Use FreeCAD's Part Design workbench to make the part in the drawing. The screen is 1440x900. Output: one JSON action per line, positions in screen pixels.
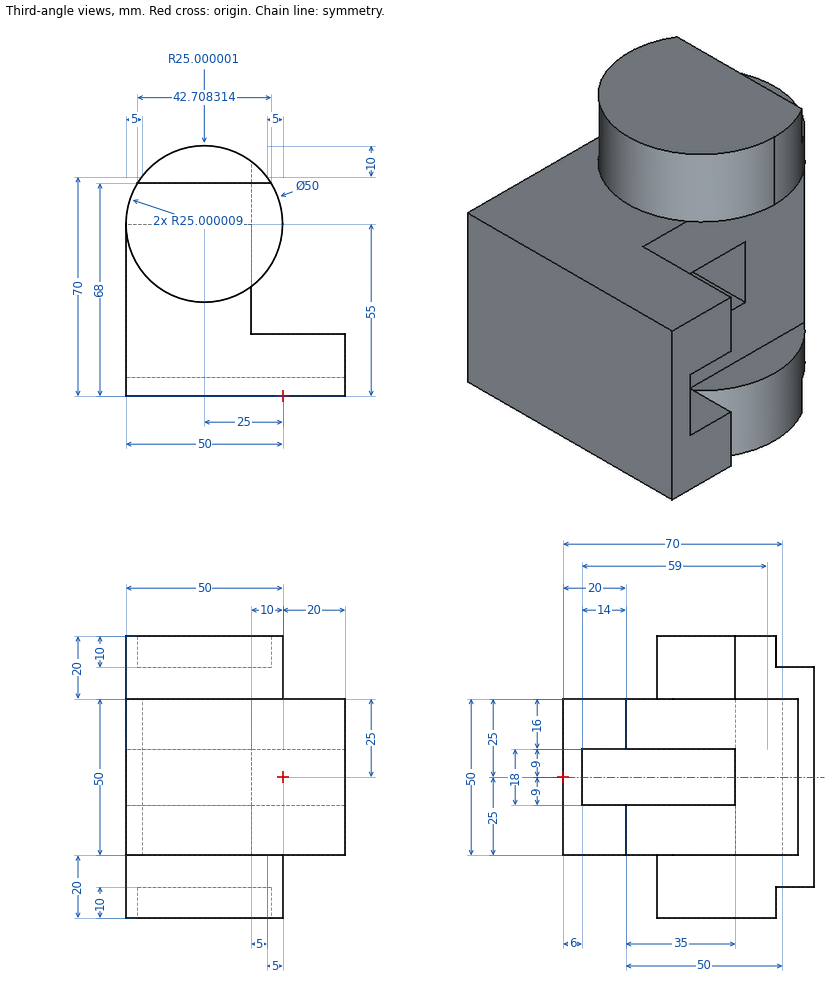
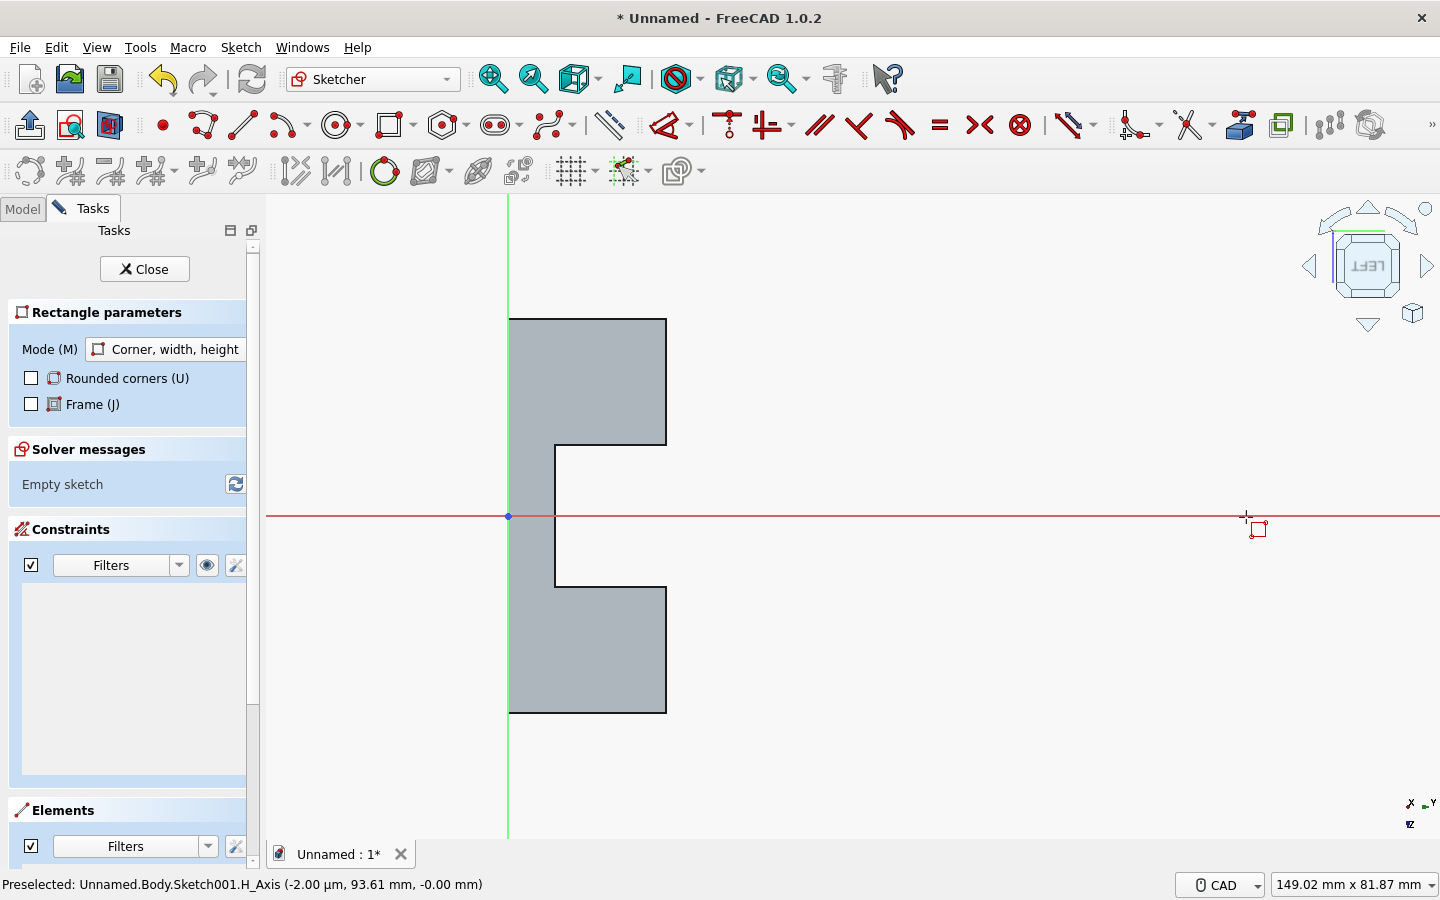
{"action": "left_click", "coordinate": [508, 319]}
{"action": "mouse_move", "coordinate": [1060, 713]}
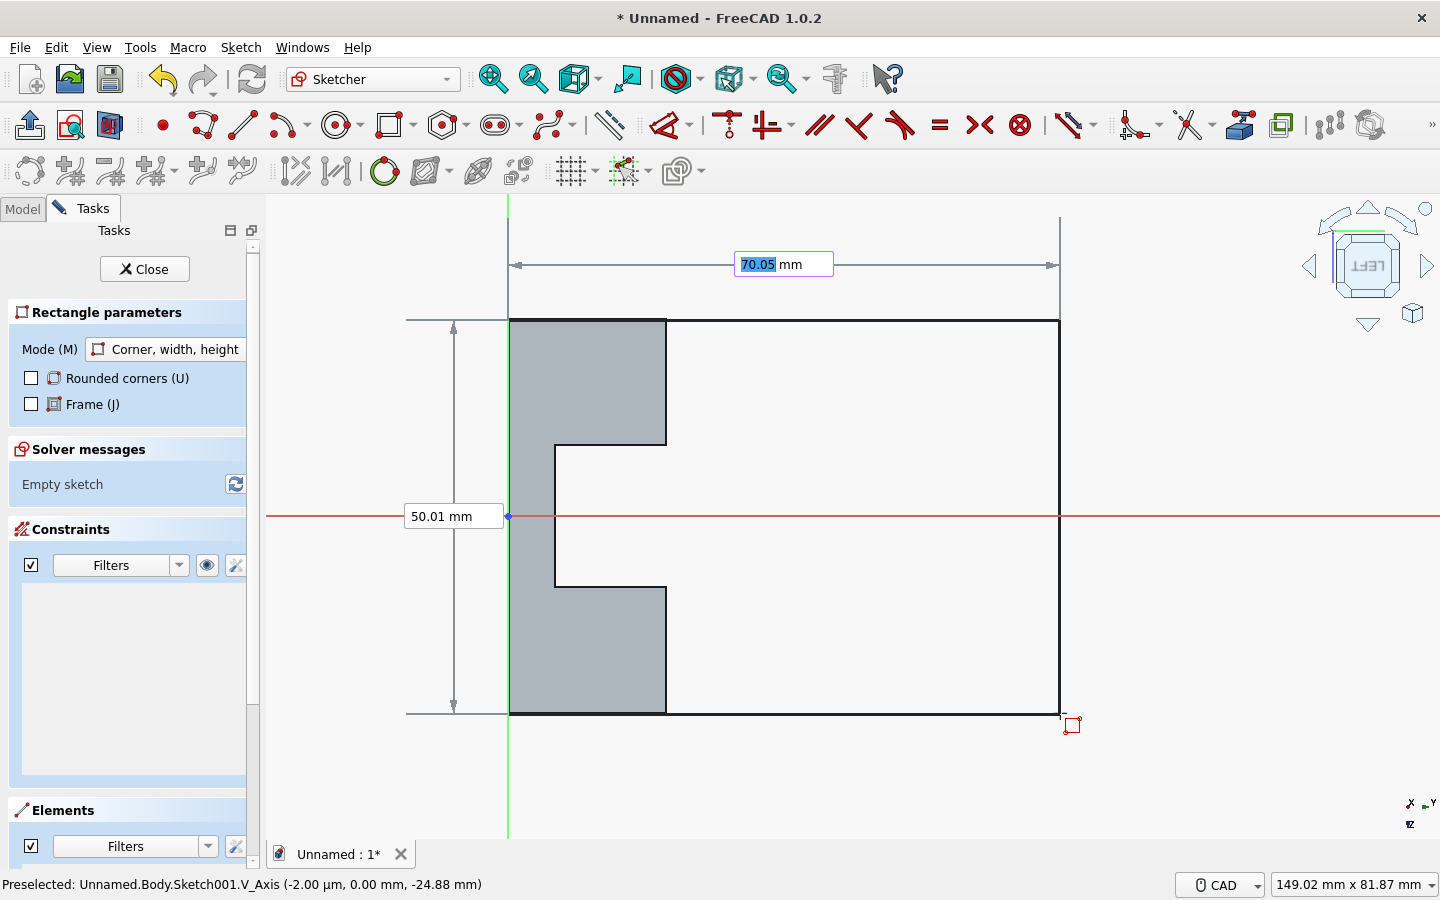
{"action": "type", "text": "70"}
{"action": "key", "text": "Tab"}
{"action": "type", "text": "50"}
{"action": "key", "text": "Return"}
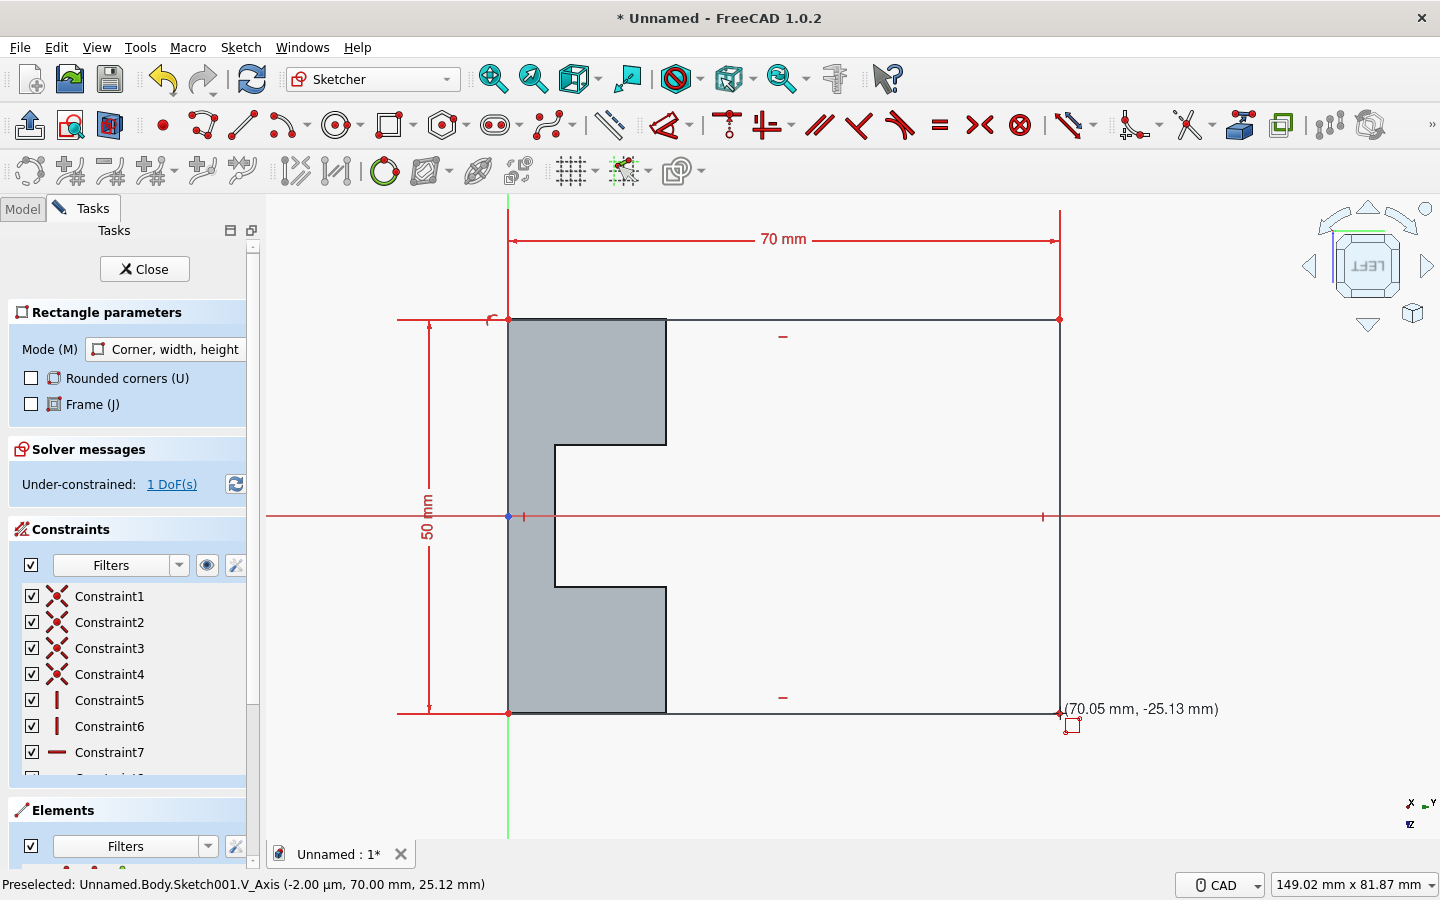
{"action": "left_click", "coordinate": [555, 445]}
{"action": "mouse_move", "coordinate": [1020, 587]}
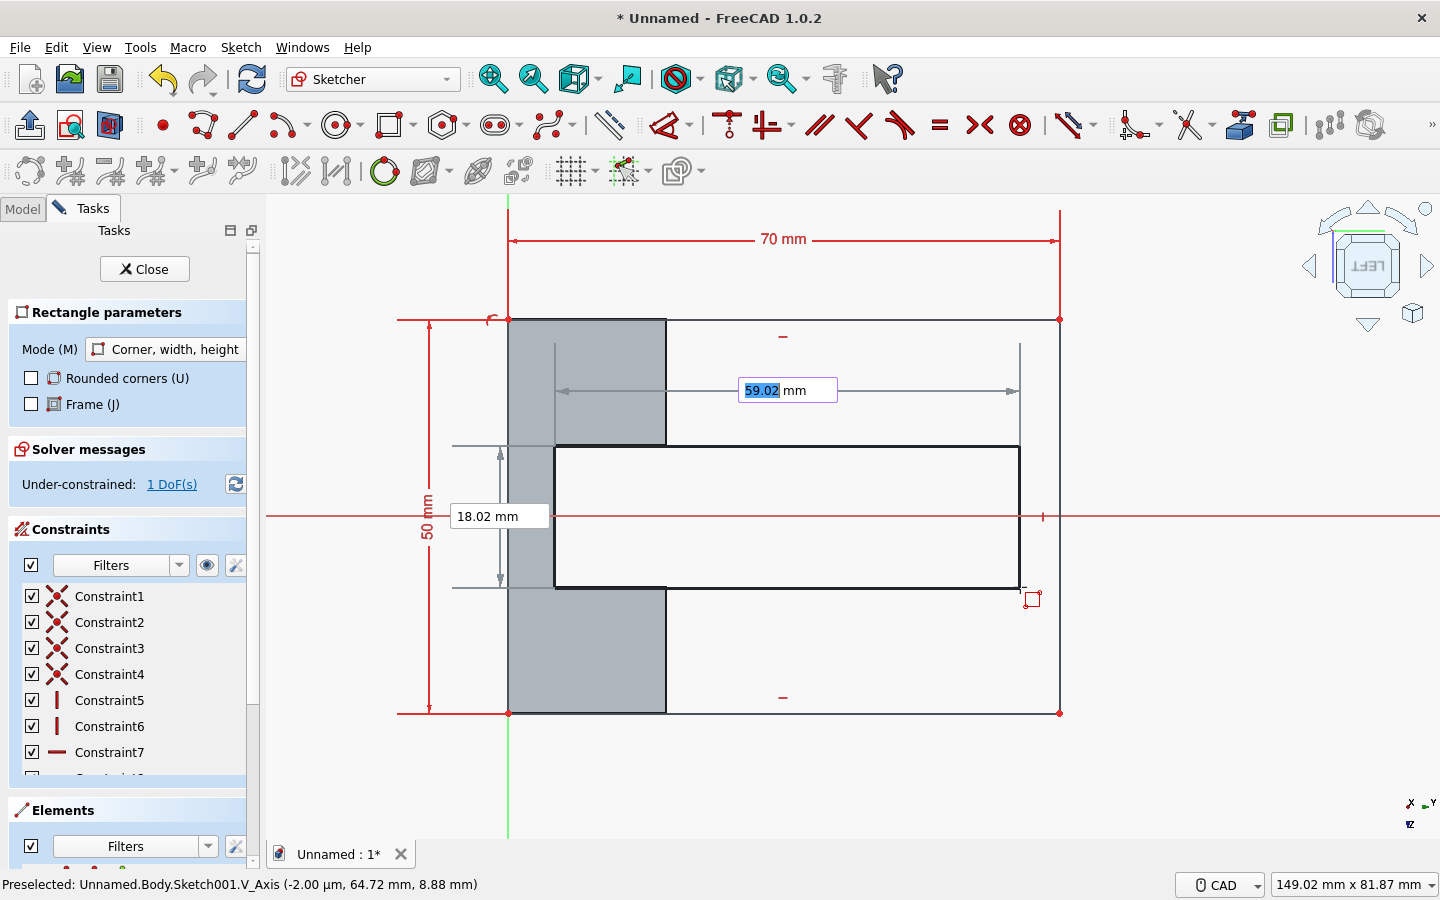
{"action": "type", "text": "59"}
{"action": "key", "text": "Tab"}
{"action": "type", "text": "18"}
{"action": "key", "text": "Return"}
{"action": "key", "text": "Escape"}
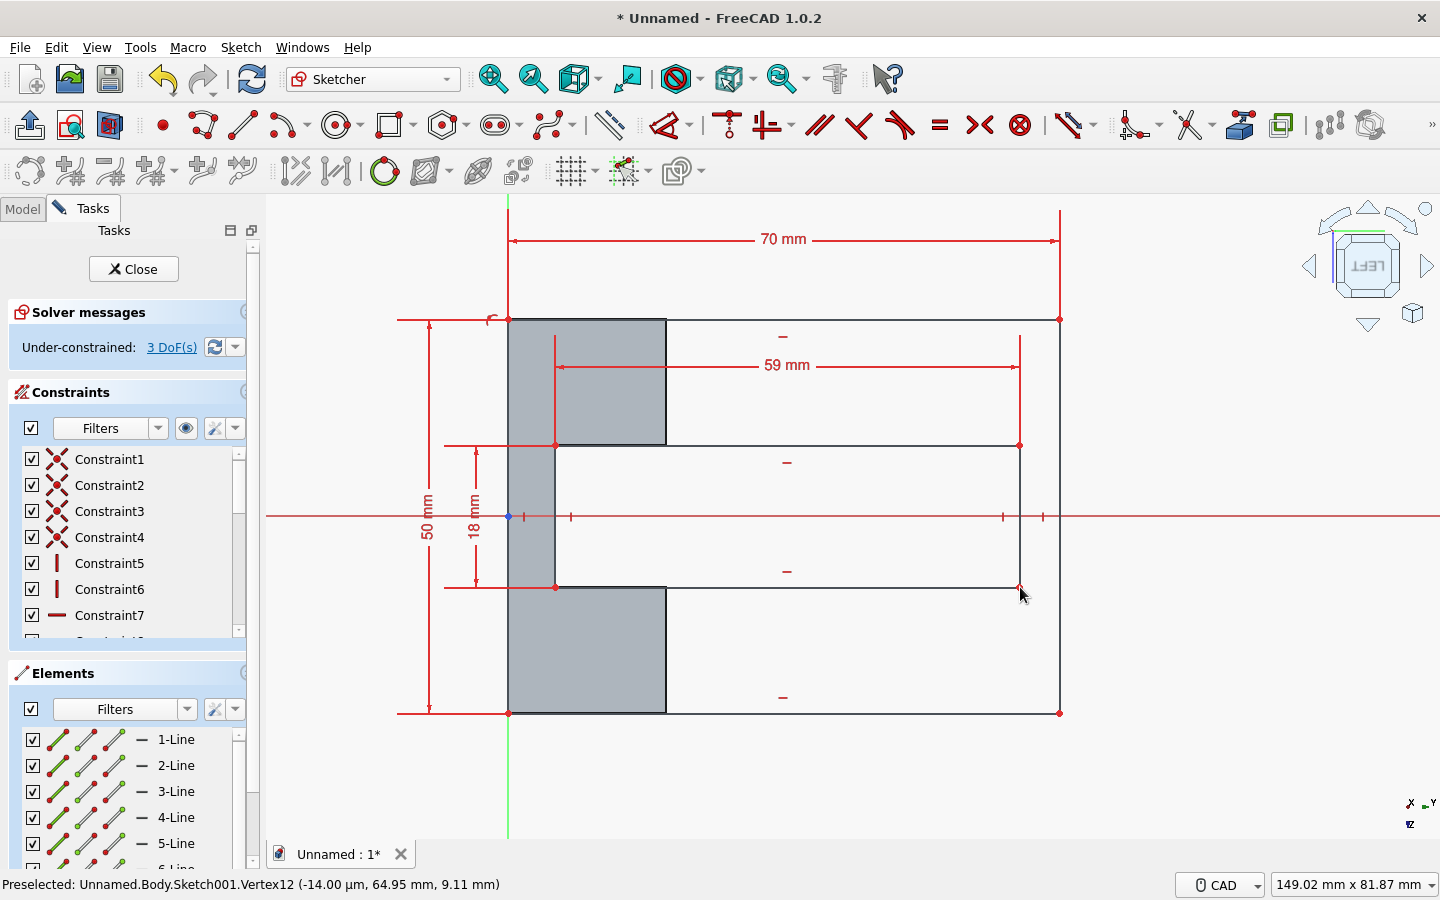
{"action": "left_click", "coordinate": [664, 126]}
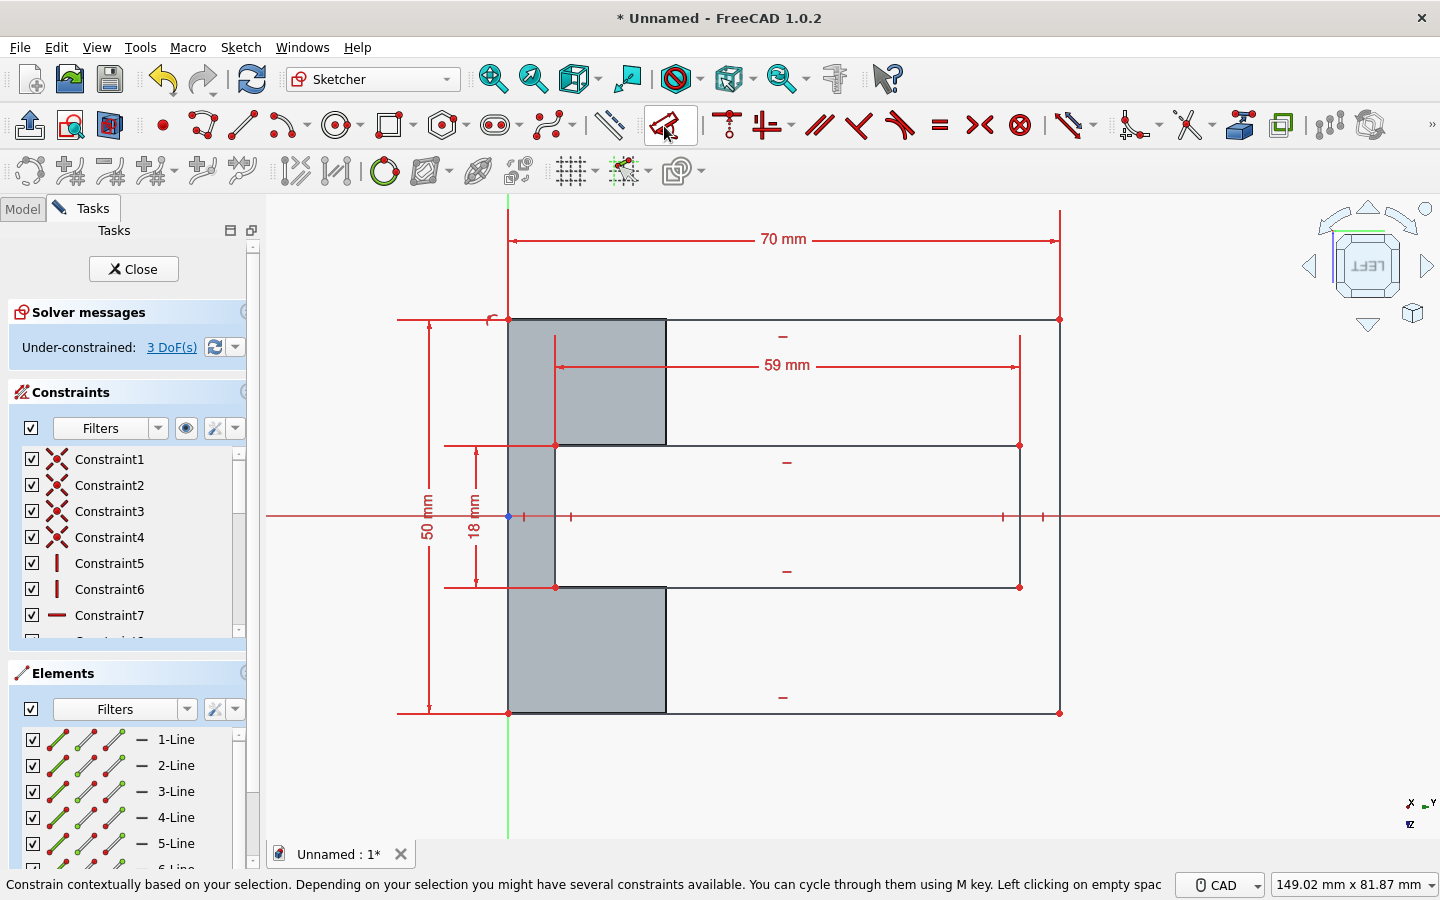
{"action": "left_click", "coordinate": [555, 446]}
{"action": "left_click", "coordinate": [532, 412]}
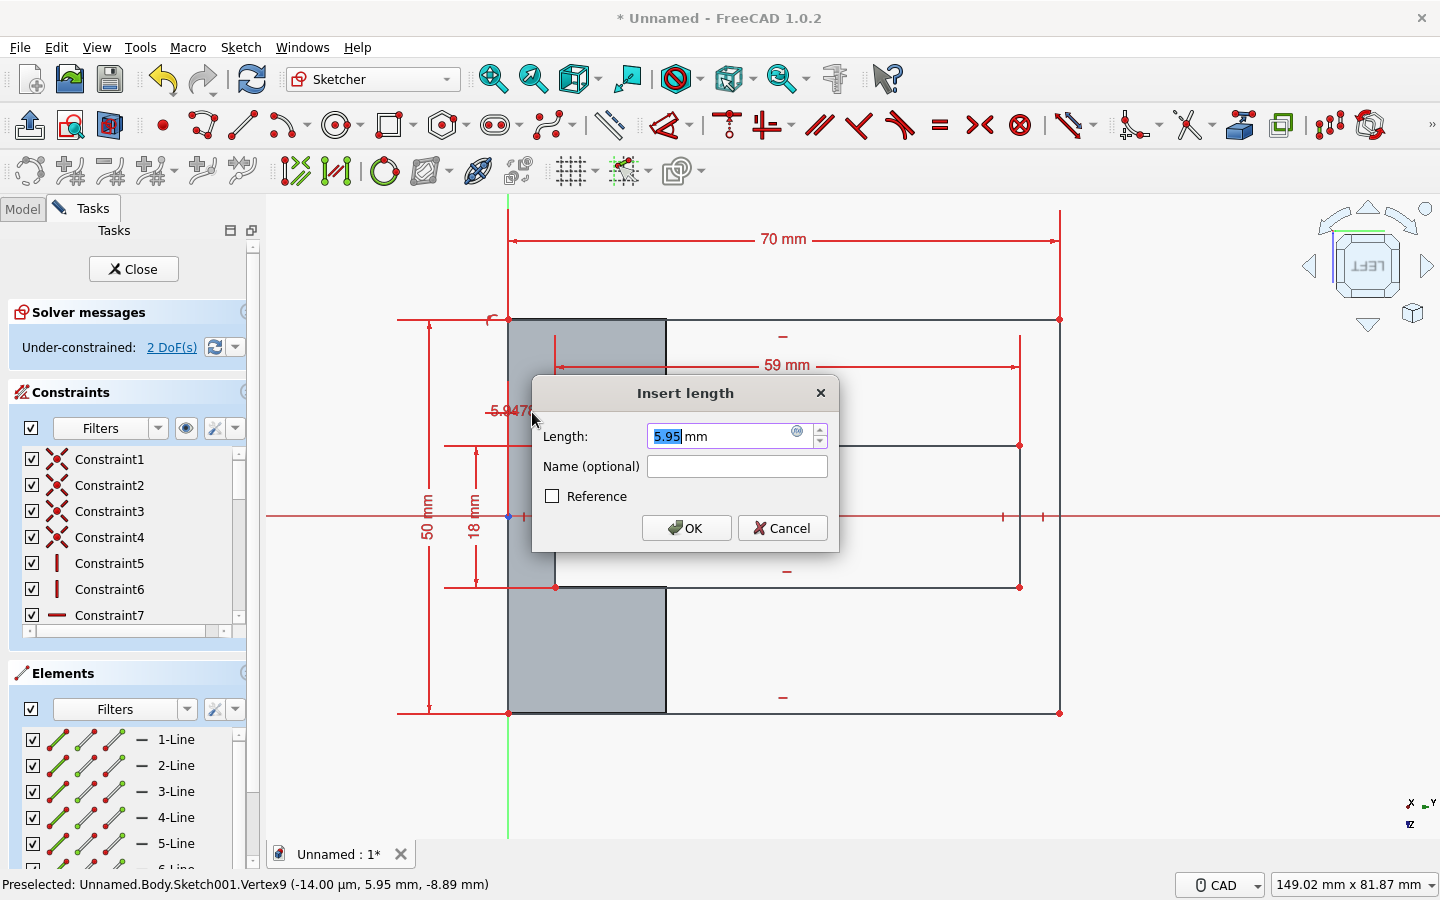
{"action": "type", "text": "6"}
{"action": "key", "text": "Return"}